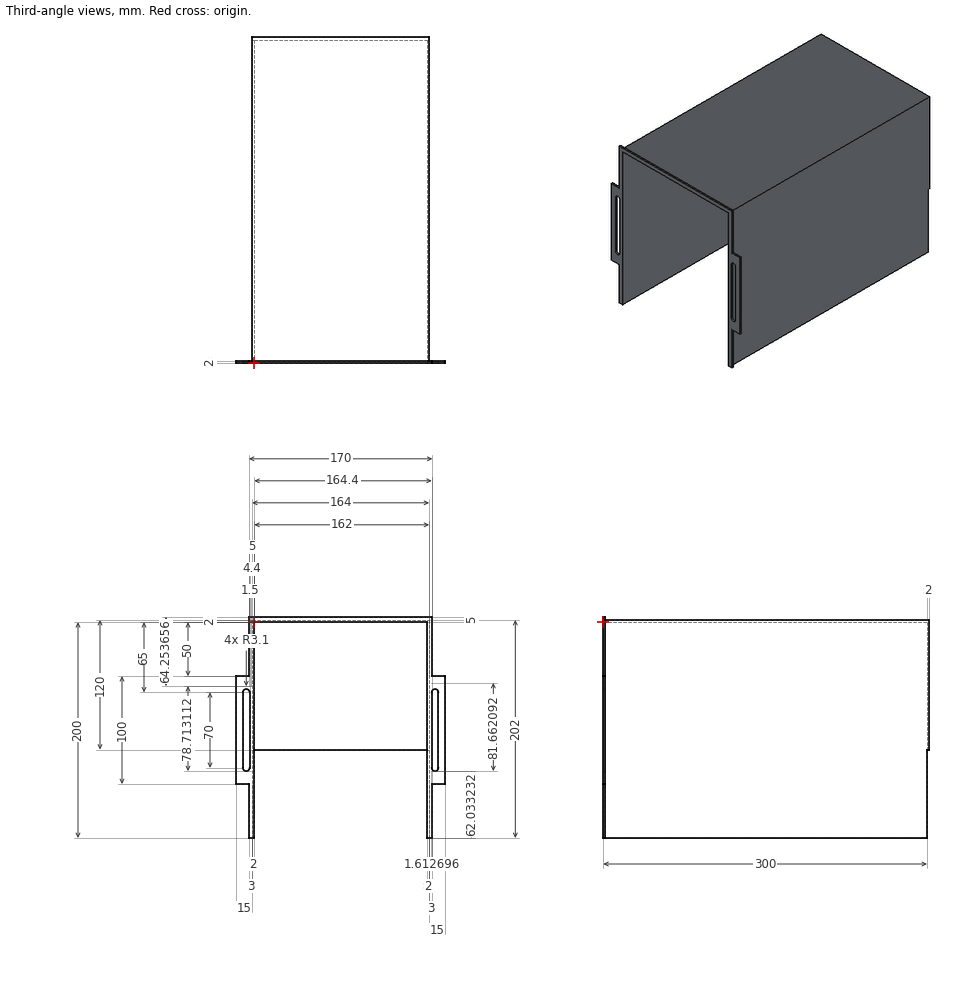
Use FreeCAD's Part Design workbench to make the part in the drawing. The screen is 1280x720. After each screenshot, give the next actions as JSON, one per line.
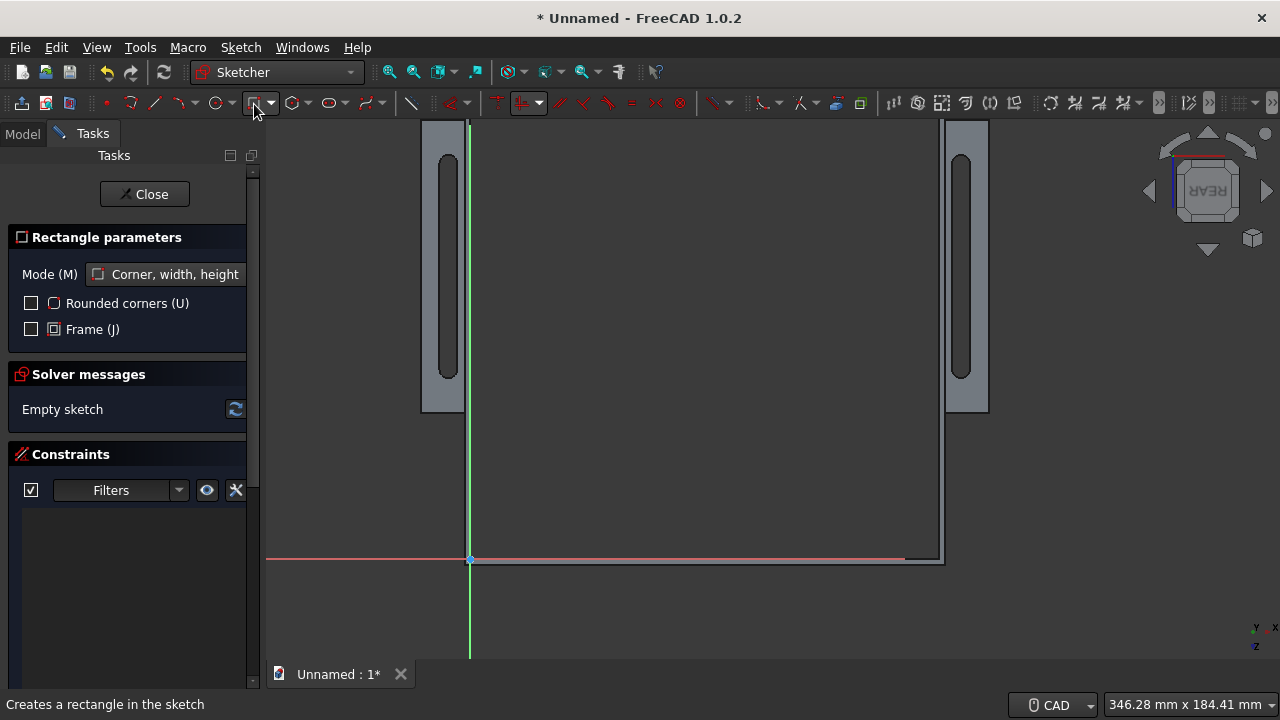
{"action": "scroll", "coordinate": [465, 214], "scroll_direction": "up", "scroll_amount": 5}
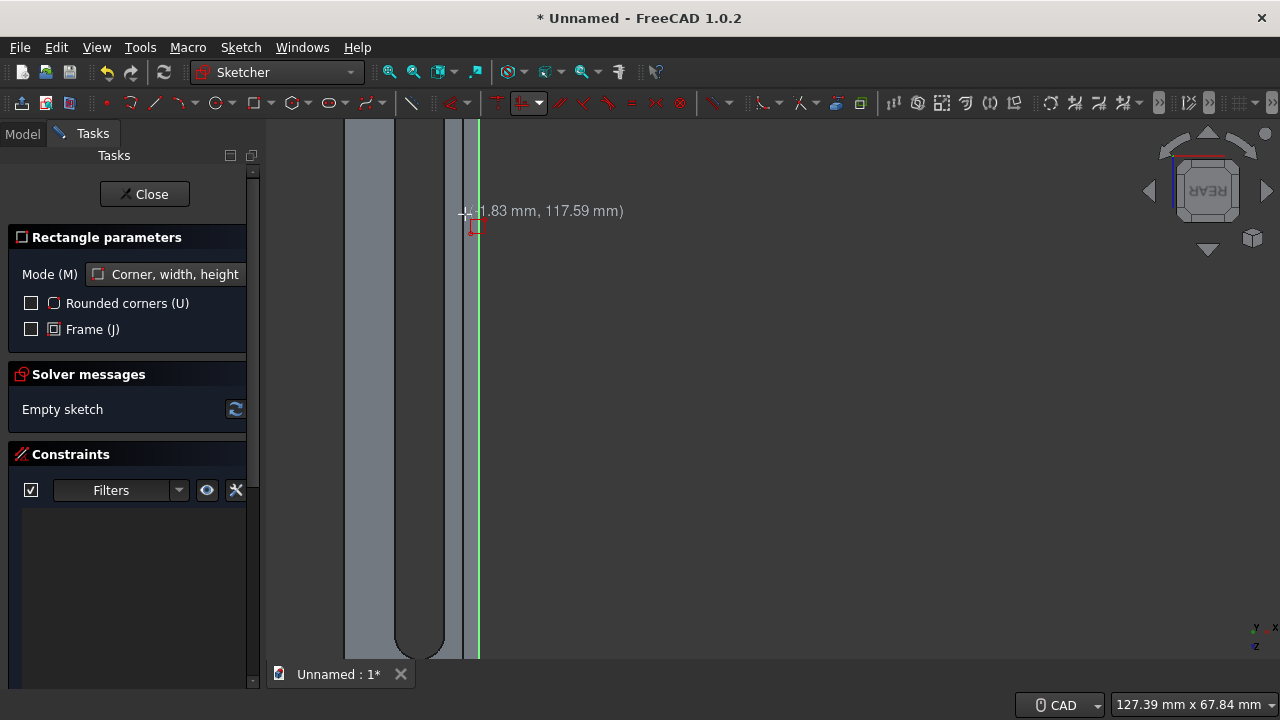
{"action": "left_click", "coordinate": [463, 213]}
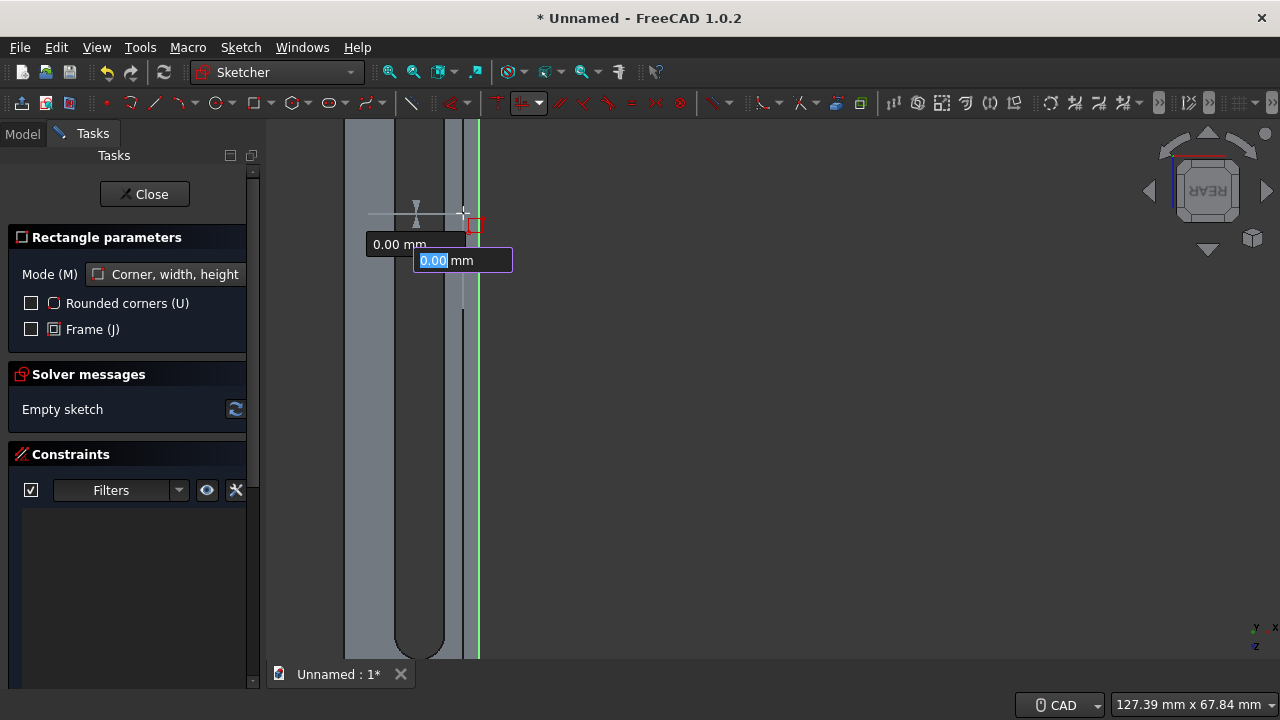
{"action": "scroll", "coordinate": [465, 213], "scroll_direction": "down", "scroll_amount": 5}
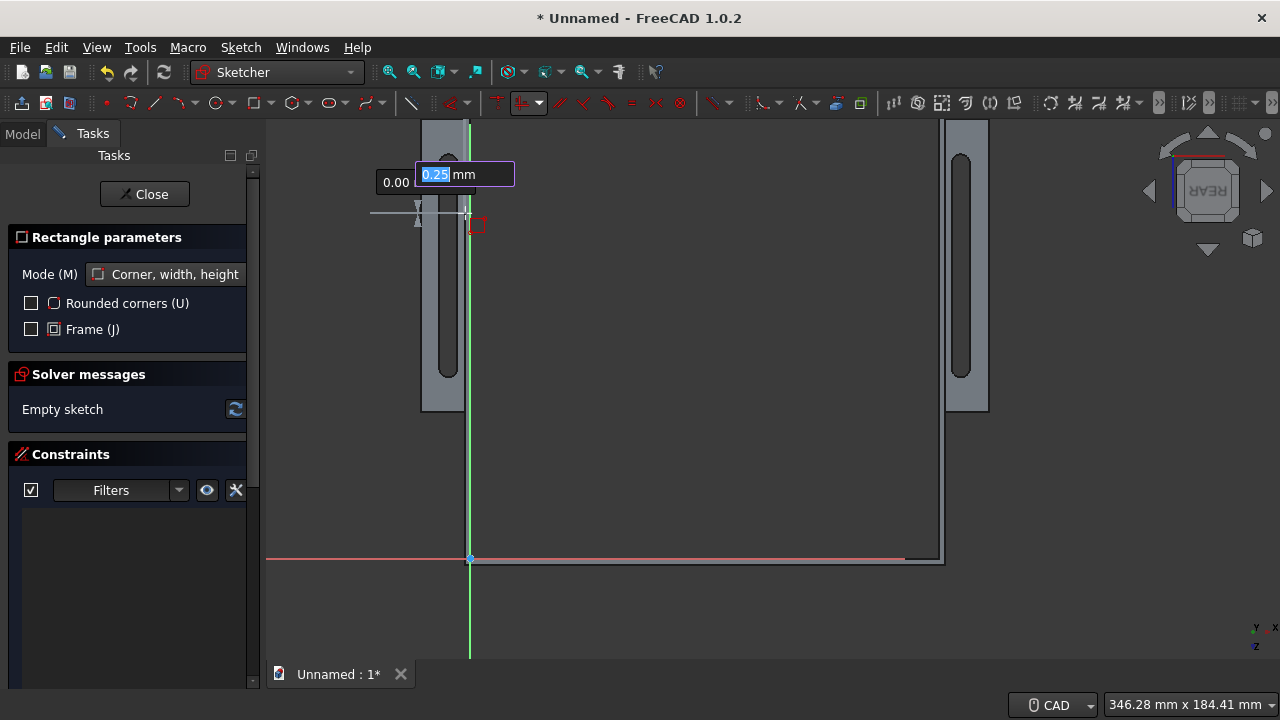
{"action": "scroll", "coordinate": [945, 565], "scroll_direction": "up", "scroll_amount": 5}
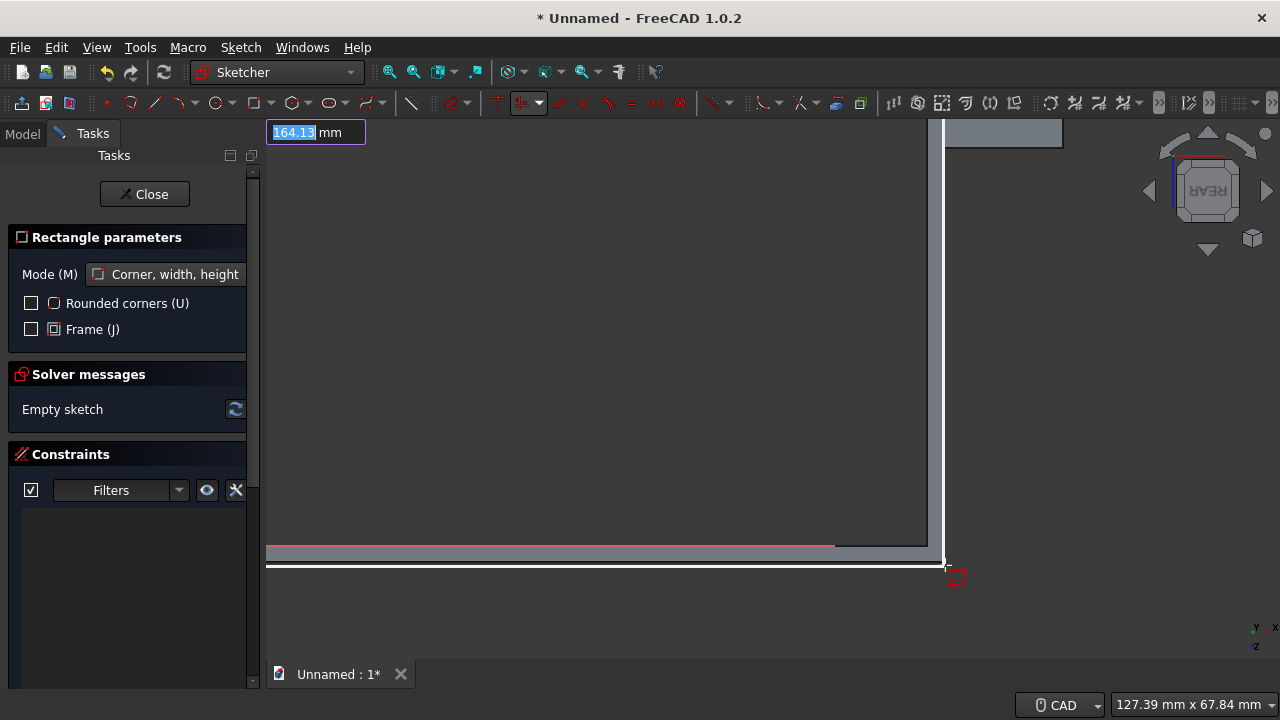
{"action": "left_click", "coordinate": [943, 562]}
{"action": "key", "text": "Escape"}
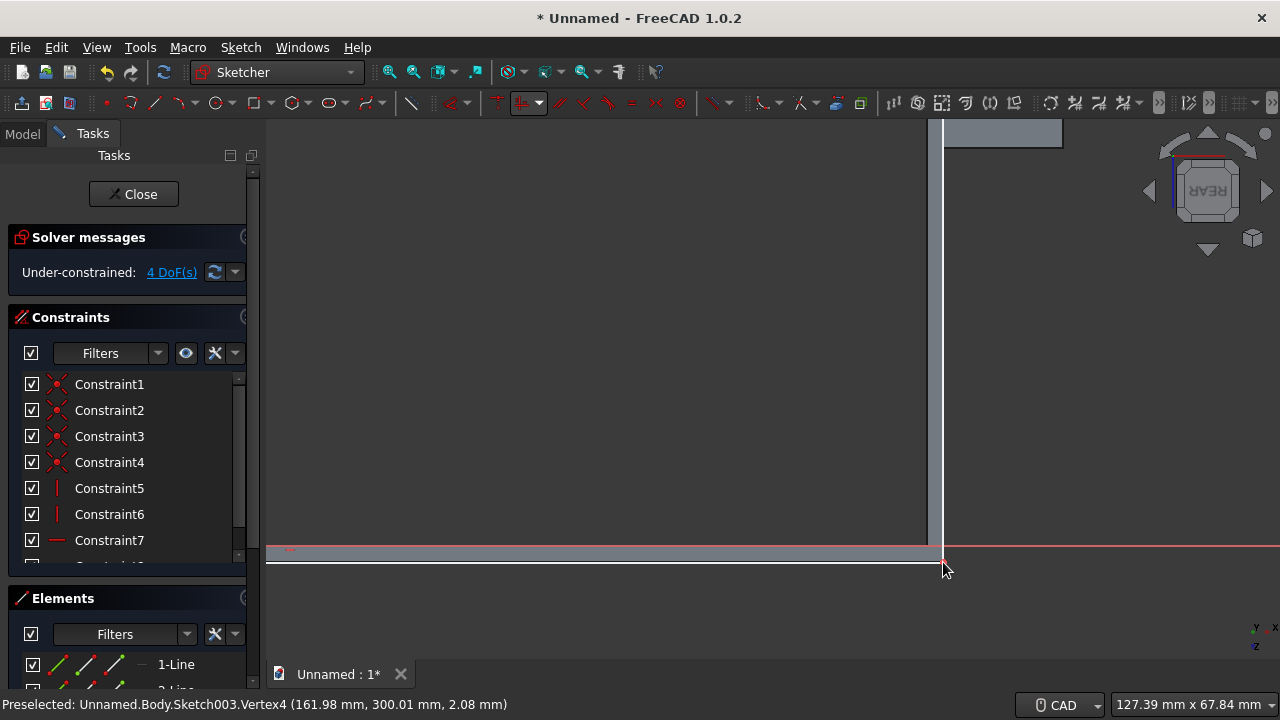
{"action": "left_click", "coordinate": [450, 104]}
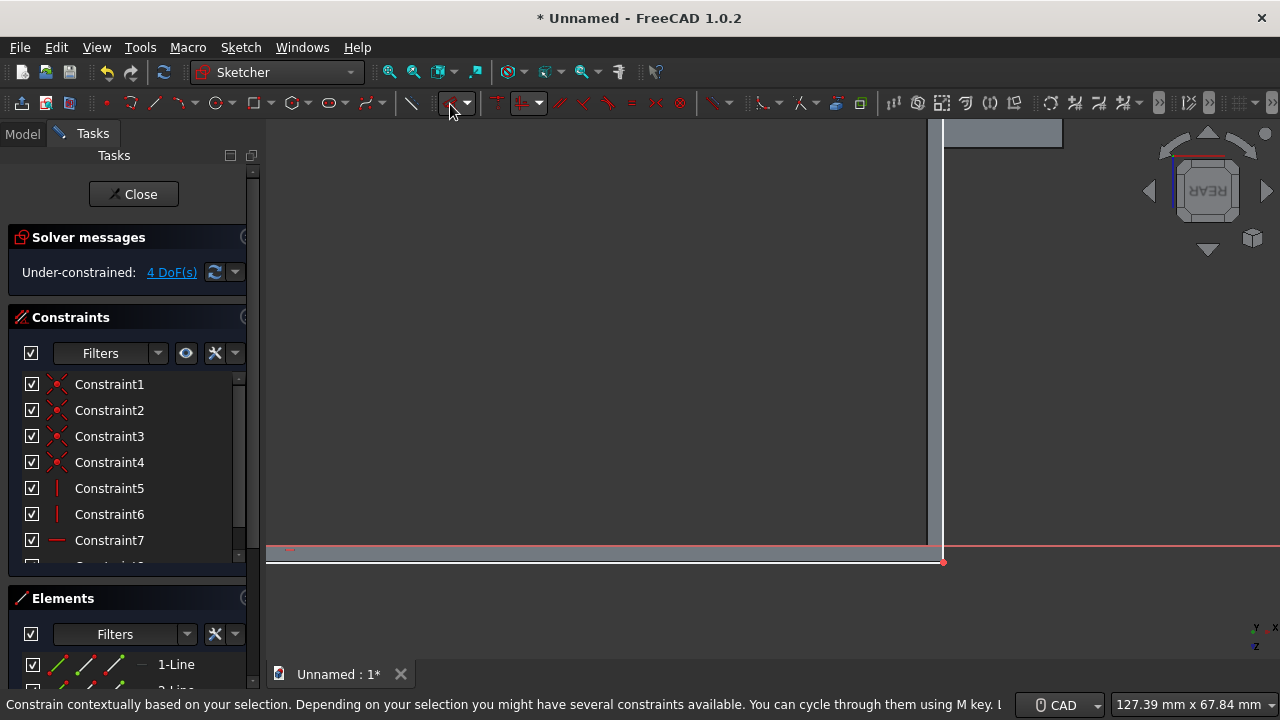
{"action": "scroll", "coordinate": [945, 566], "scroll_direction": "down", "scroll_amount": 5}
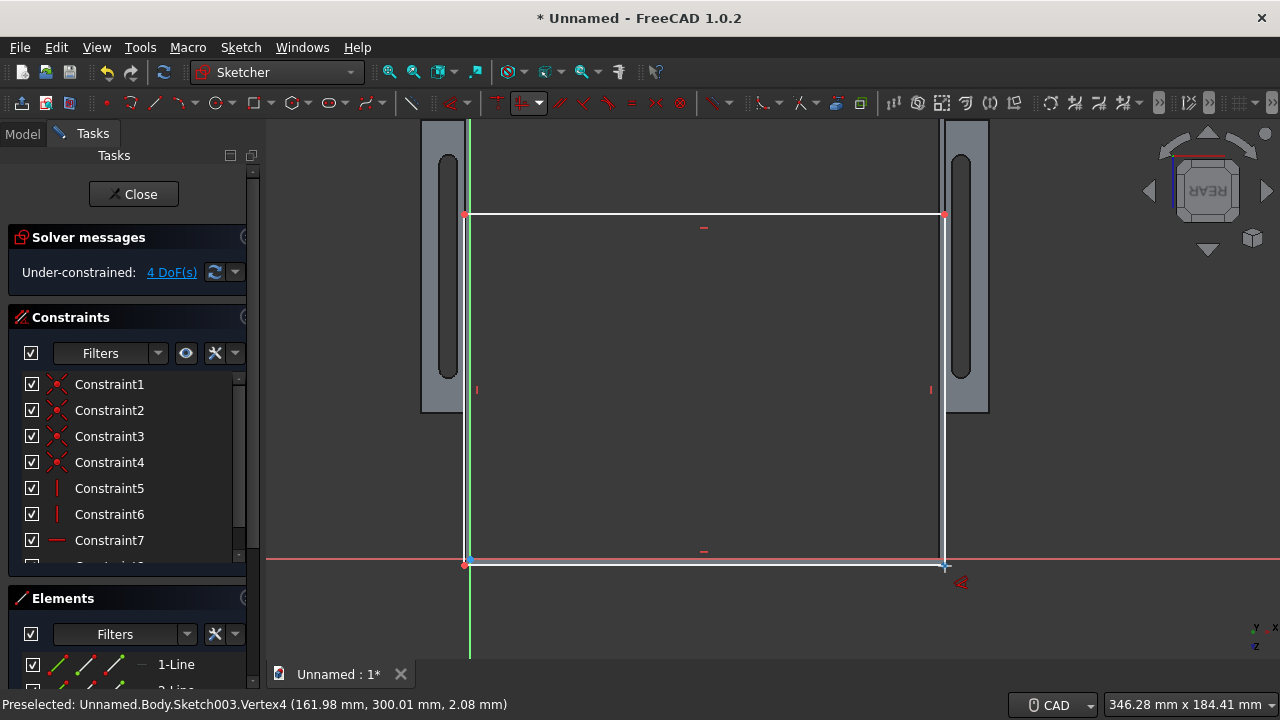
{"action": "scroll", "coordinate": [464, 214], "scroll_direction": "up", "scroll_amount": 10}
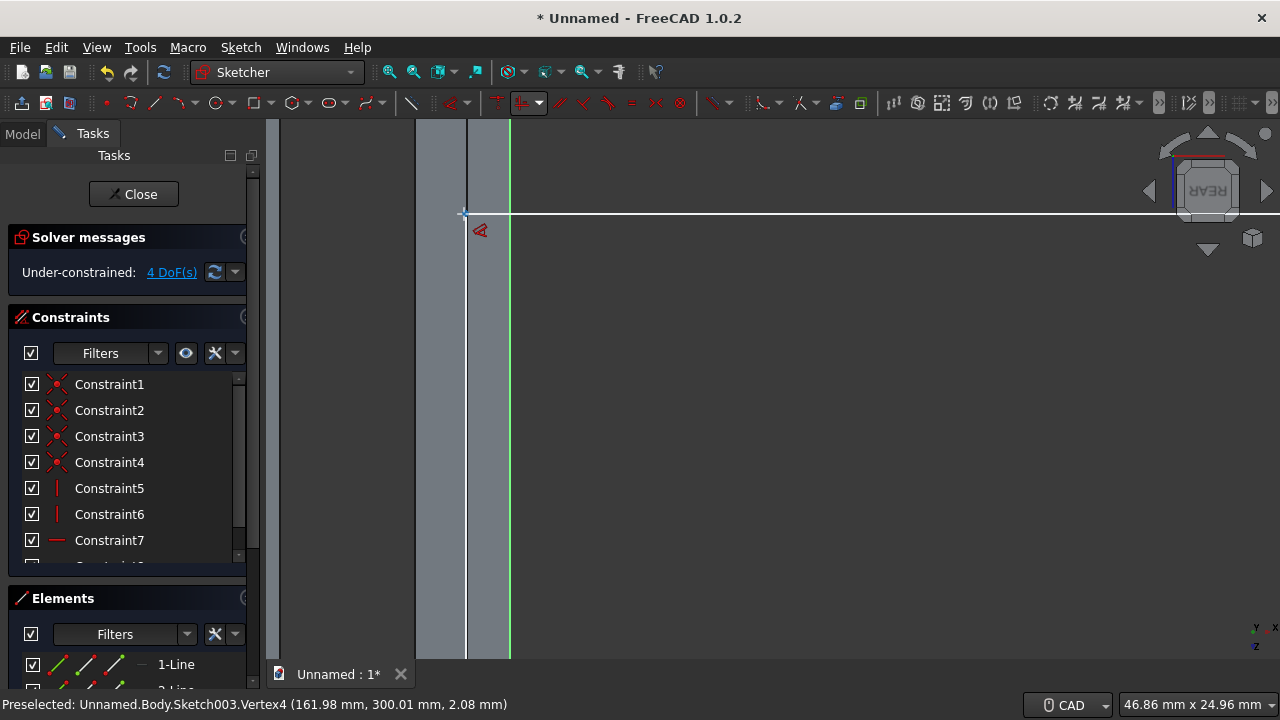
{"action": "left_click", "coordinate": [466, 214]}
{"action": "left_click", "coordinate": [488, 180]}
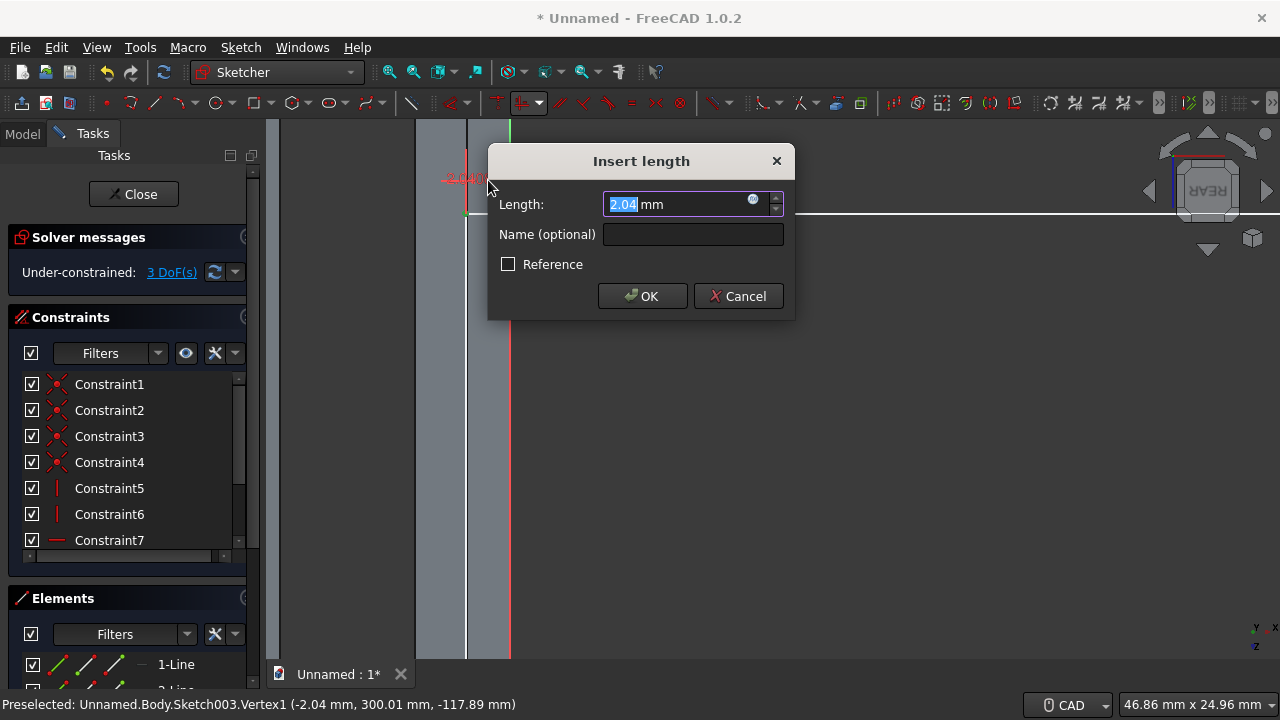
{"action": "type", "text": "2"}
{"action": "key", "text": "Return"}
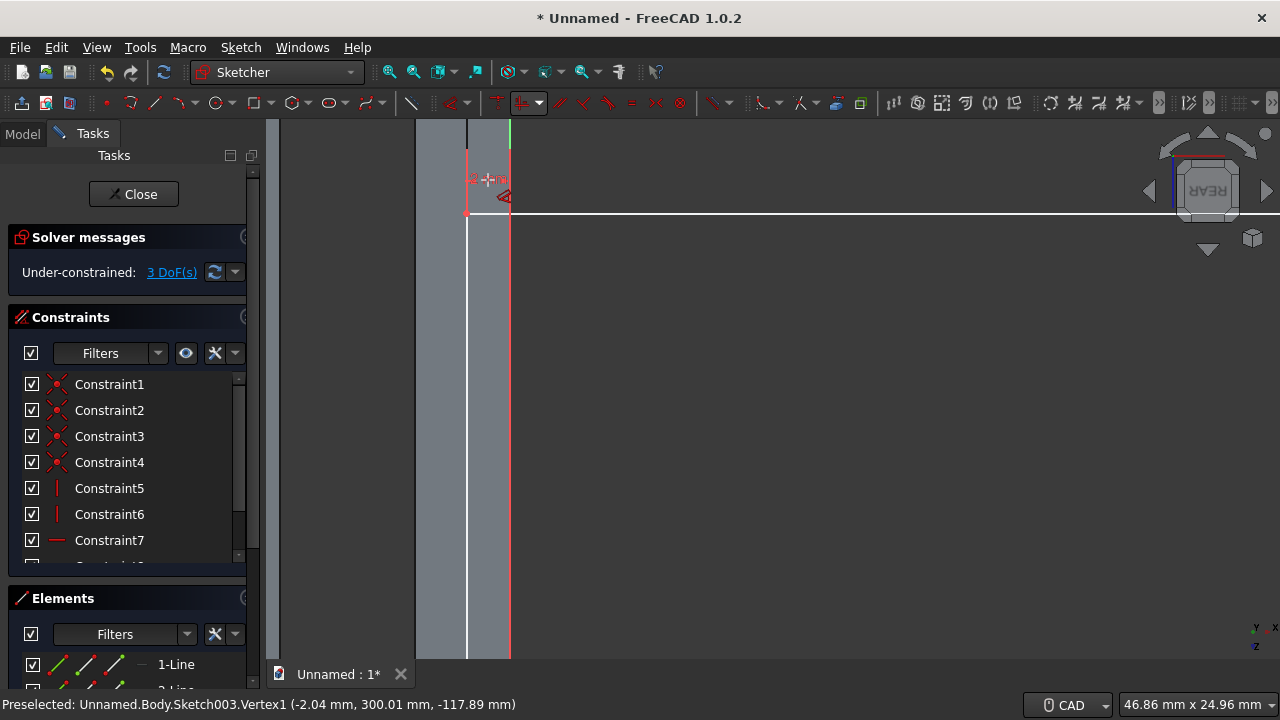
{"action": "scroll", "coordinate": [464, 214], "scroll_direction": "down", "scroll_amount": 10}